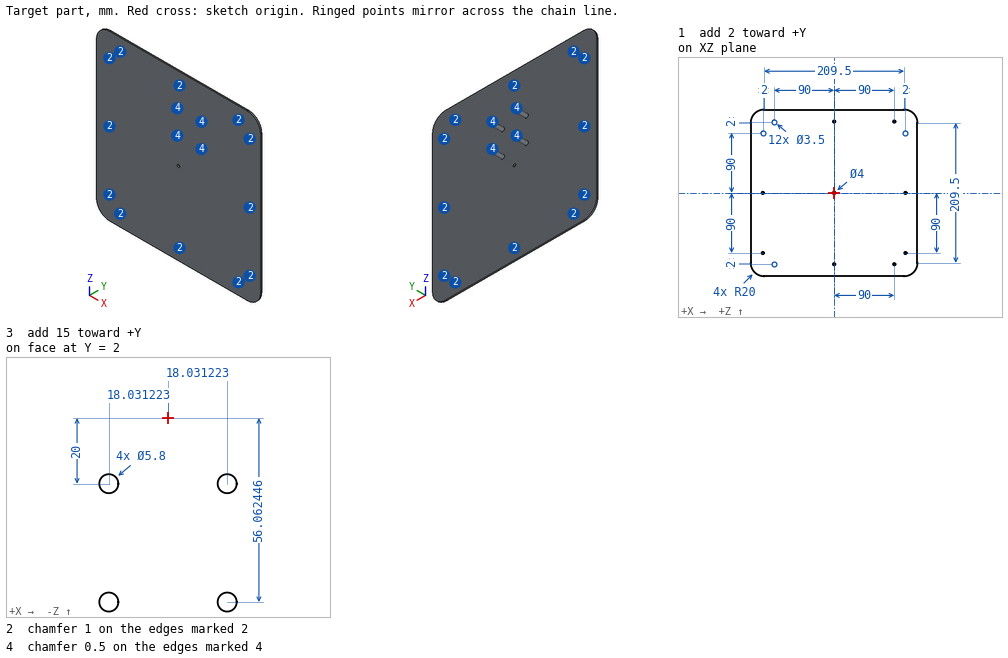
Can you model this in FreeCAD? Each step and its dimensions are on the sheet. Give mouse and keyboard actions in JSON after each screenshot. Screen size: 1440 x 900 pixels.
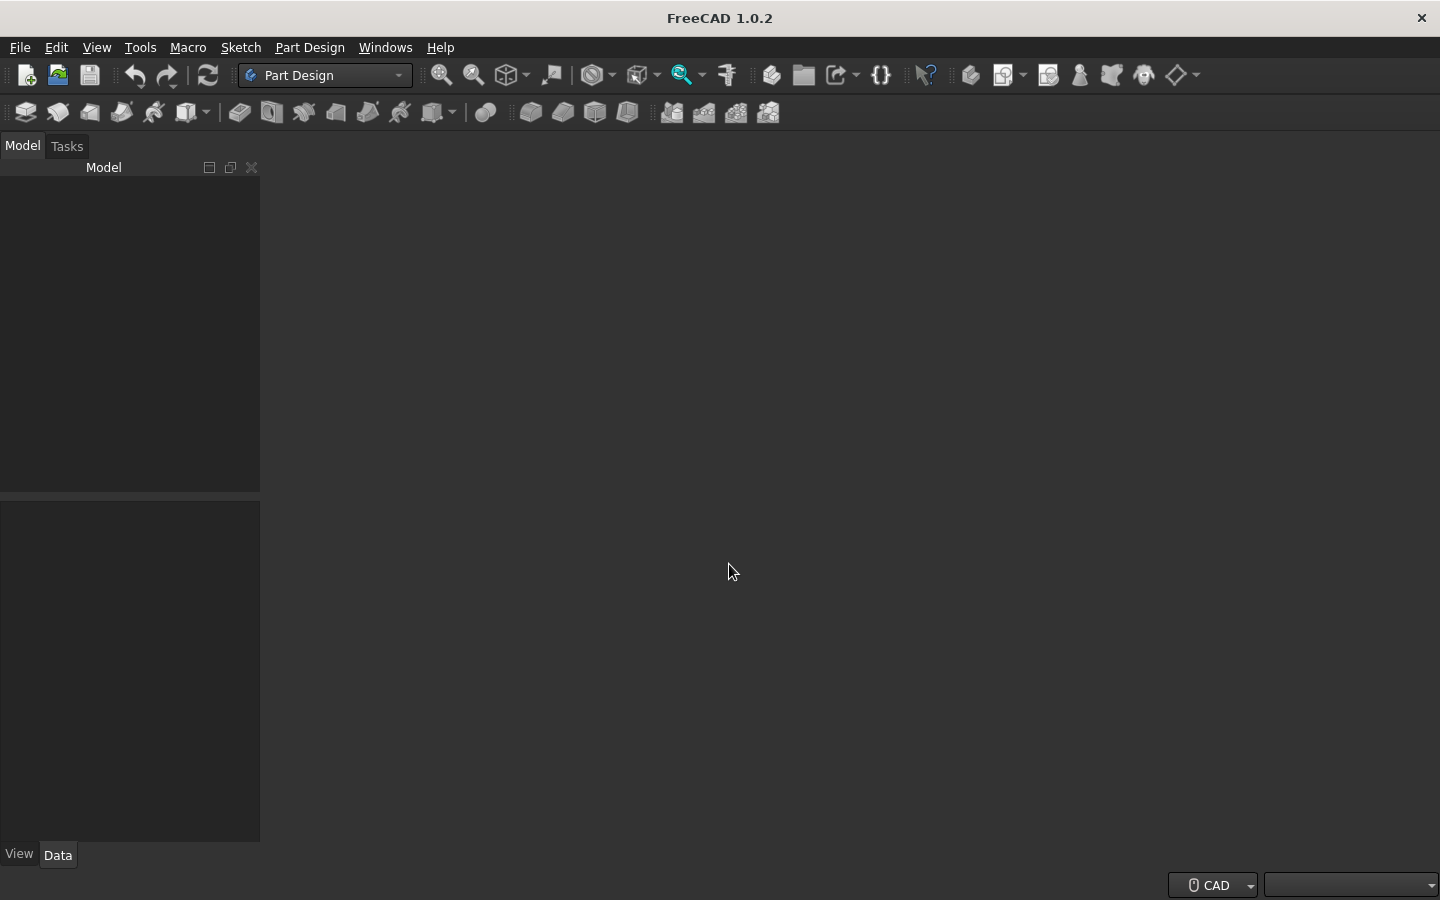
{"action": "left_click", "coordinate": [26, 76]}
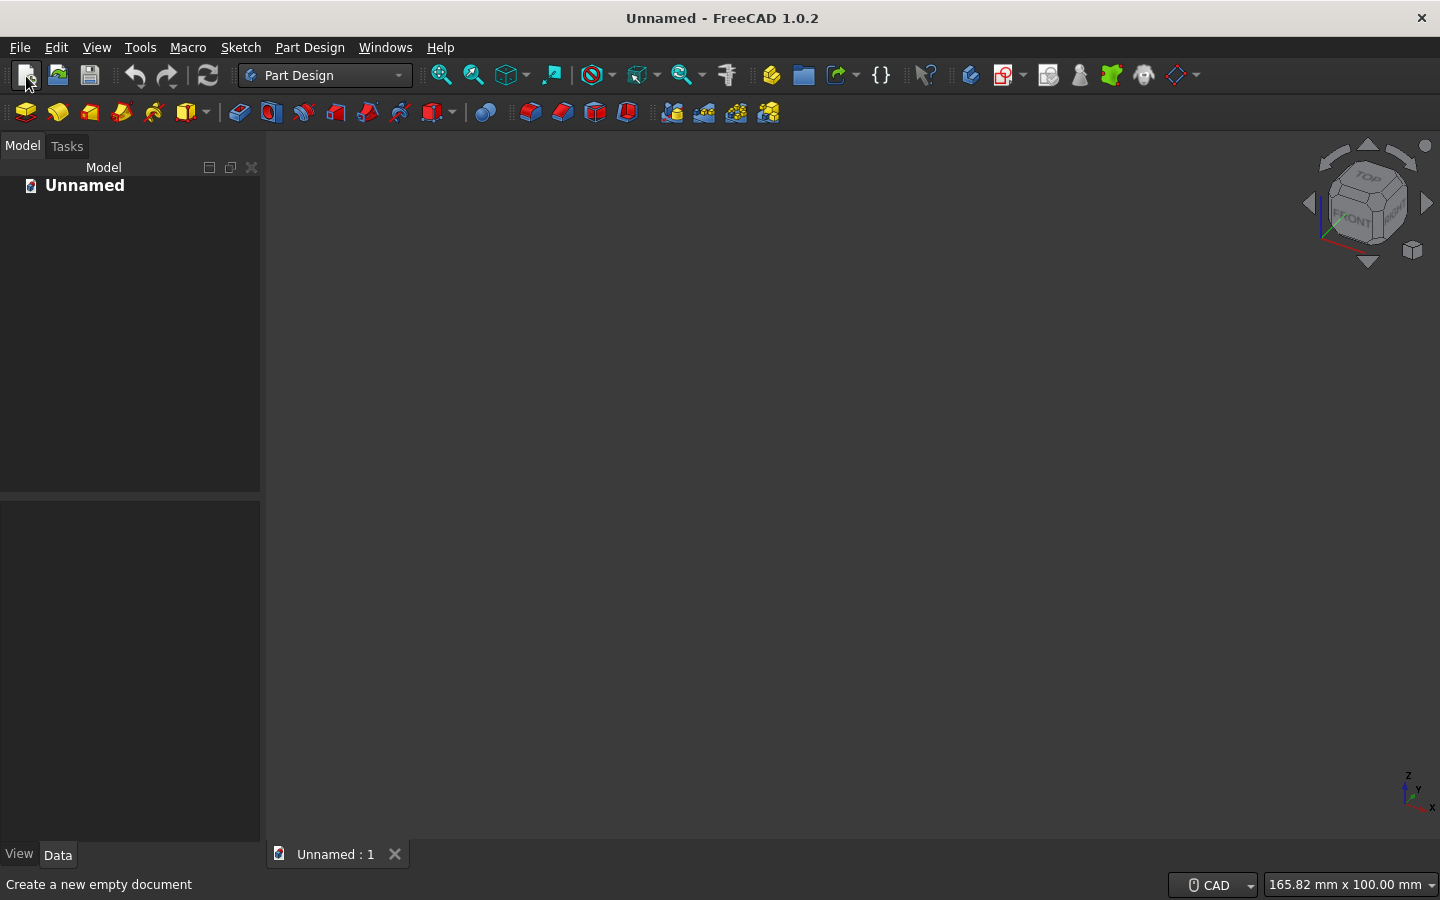
{"action": "left_click", "coordinate": [1004, 76]}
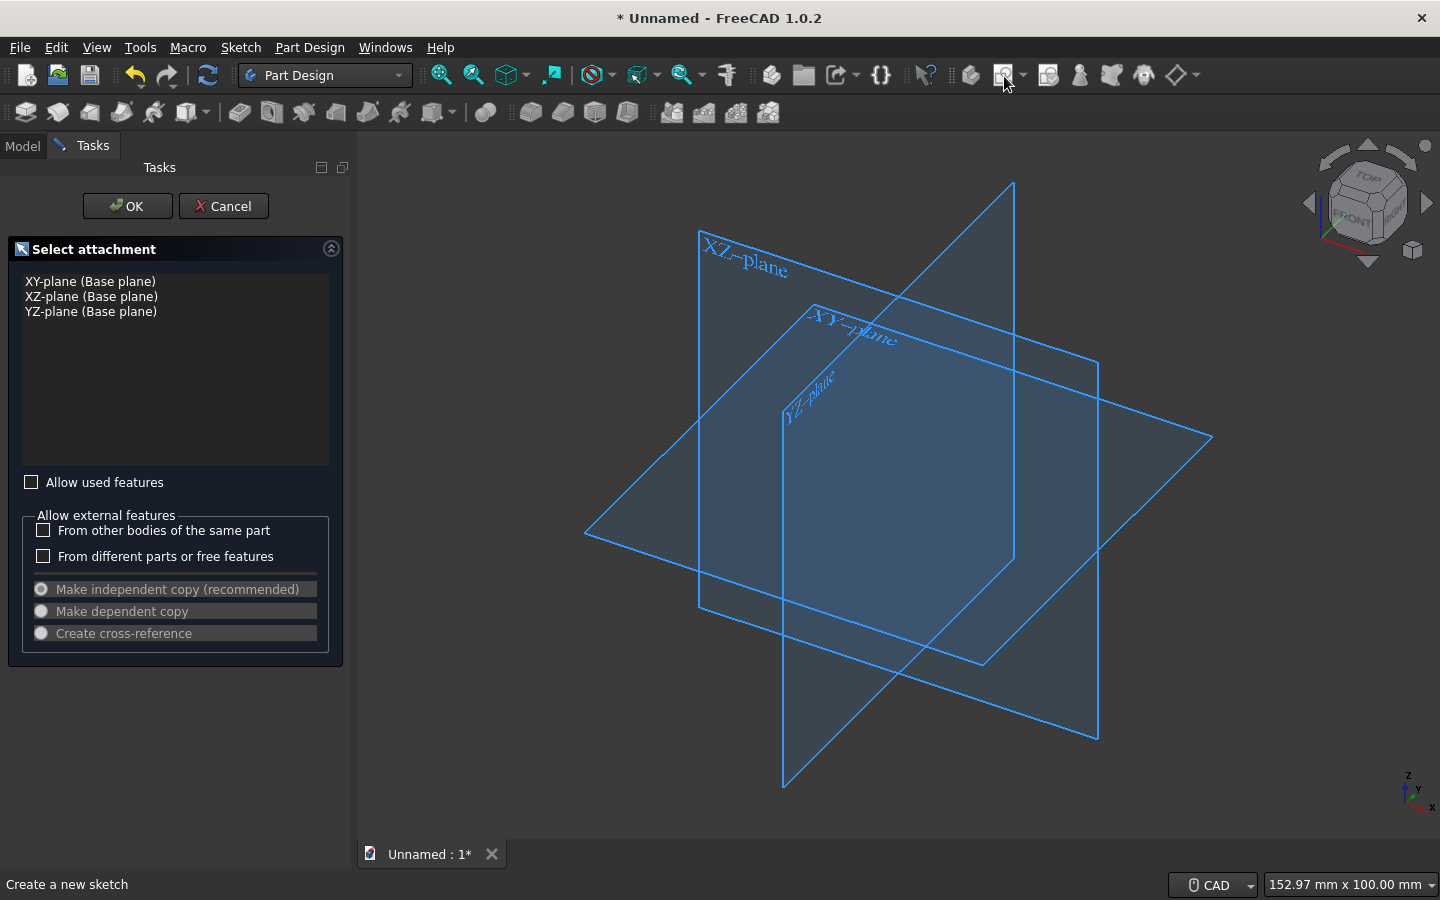
{"action": "left_click", "coordinate": [82, 296]}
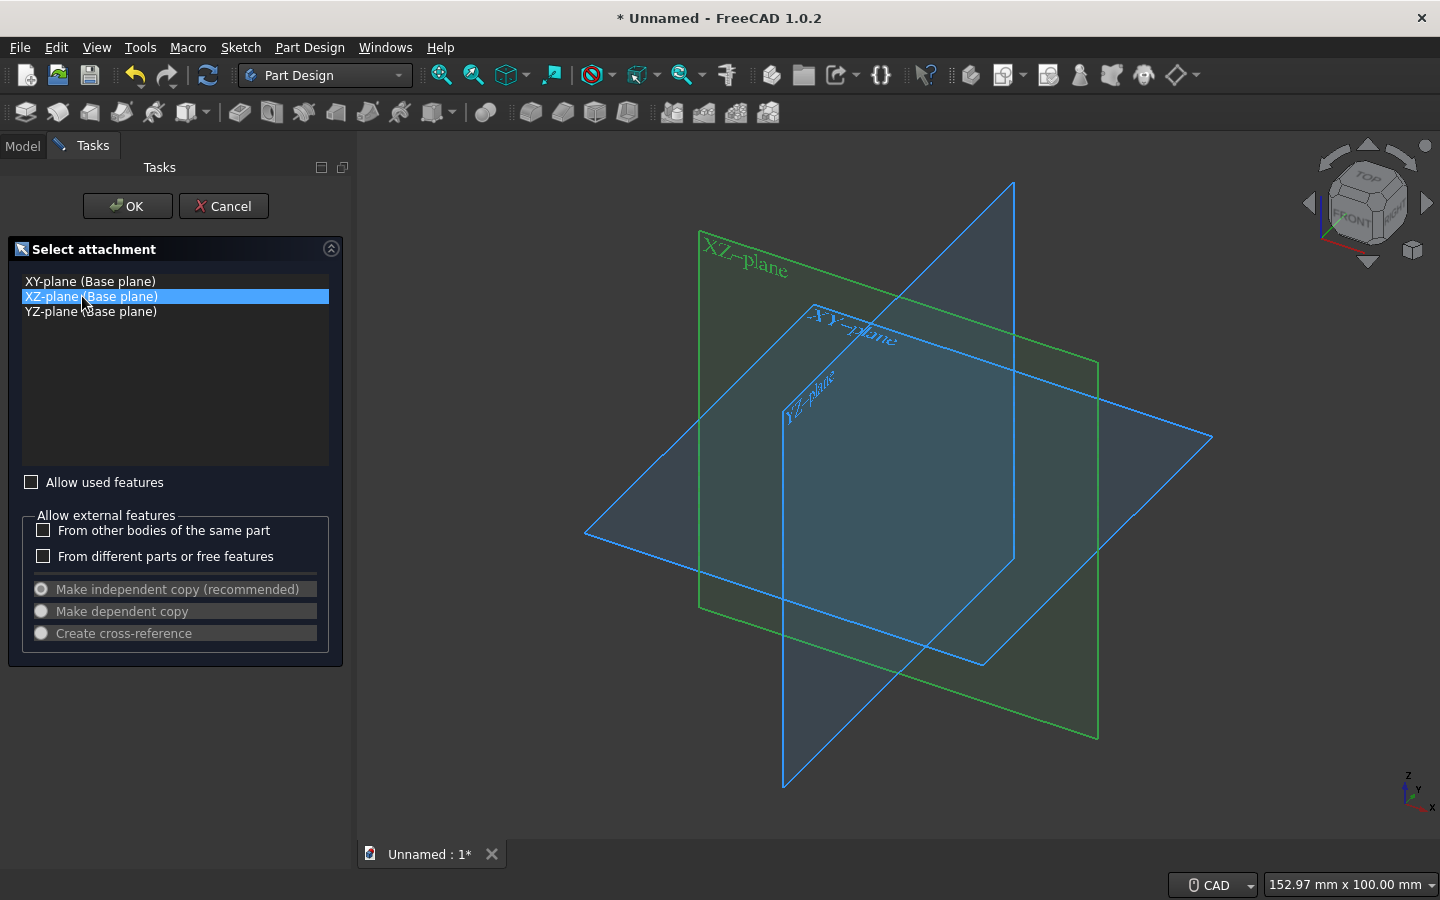
{"action": "left_click", "coordinate": [128, 206]}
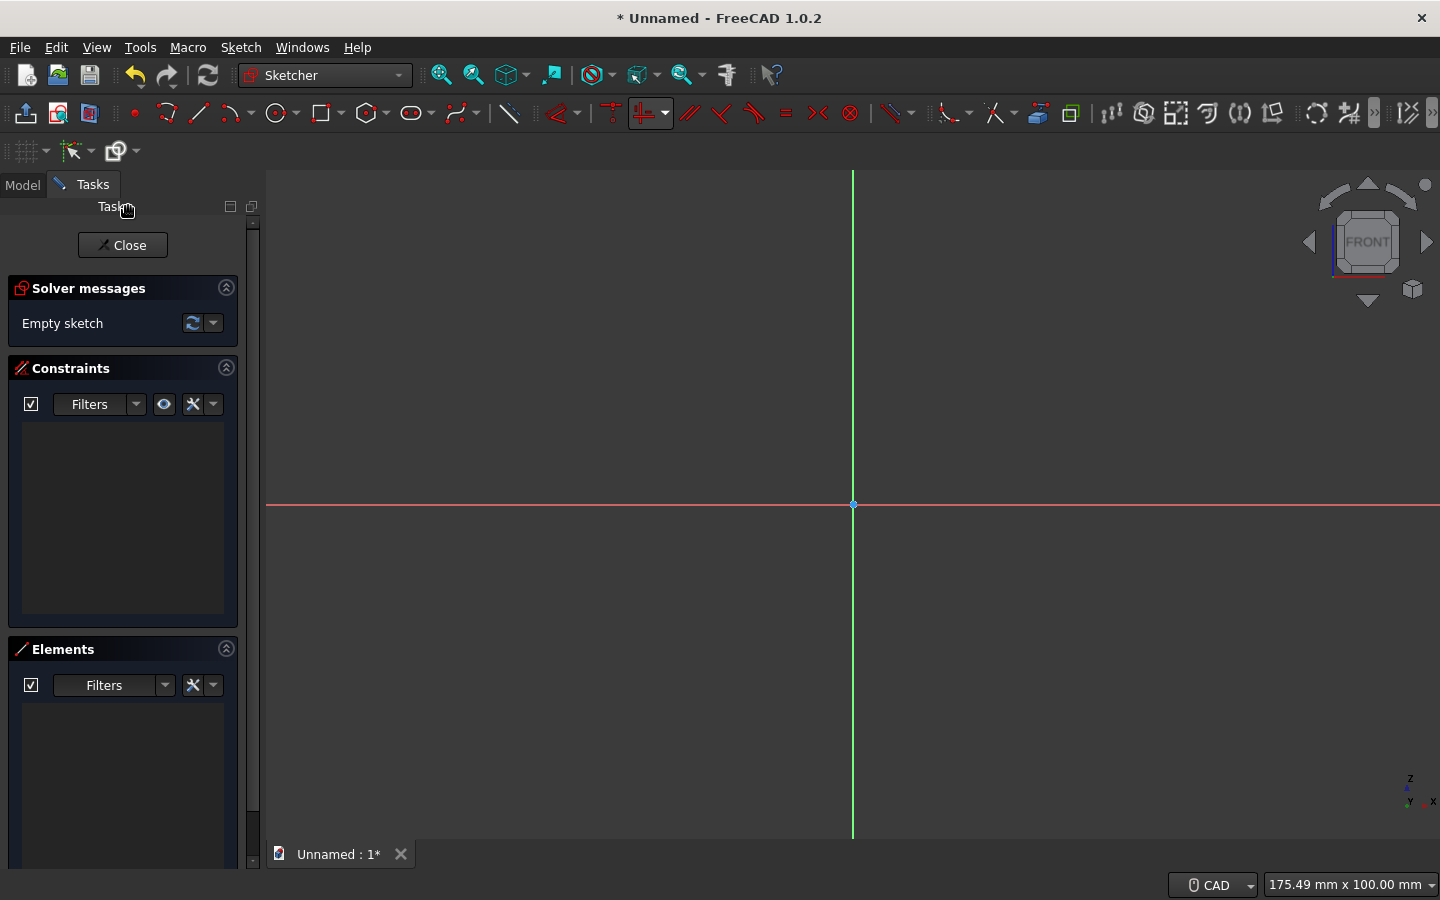
{"action": "scroll", "coordinate": [762, 504], "scroll_direction": "down", "scroll_amount": 7}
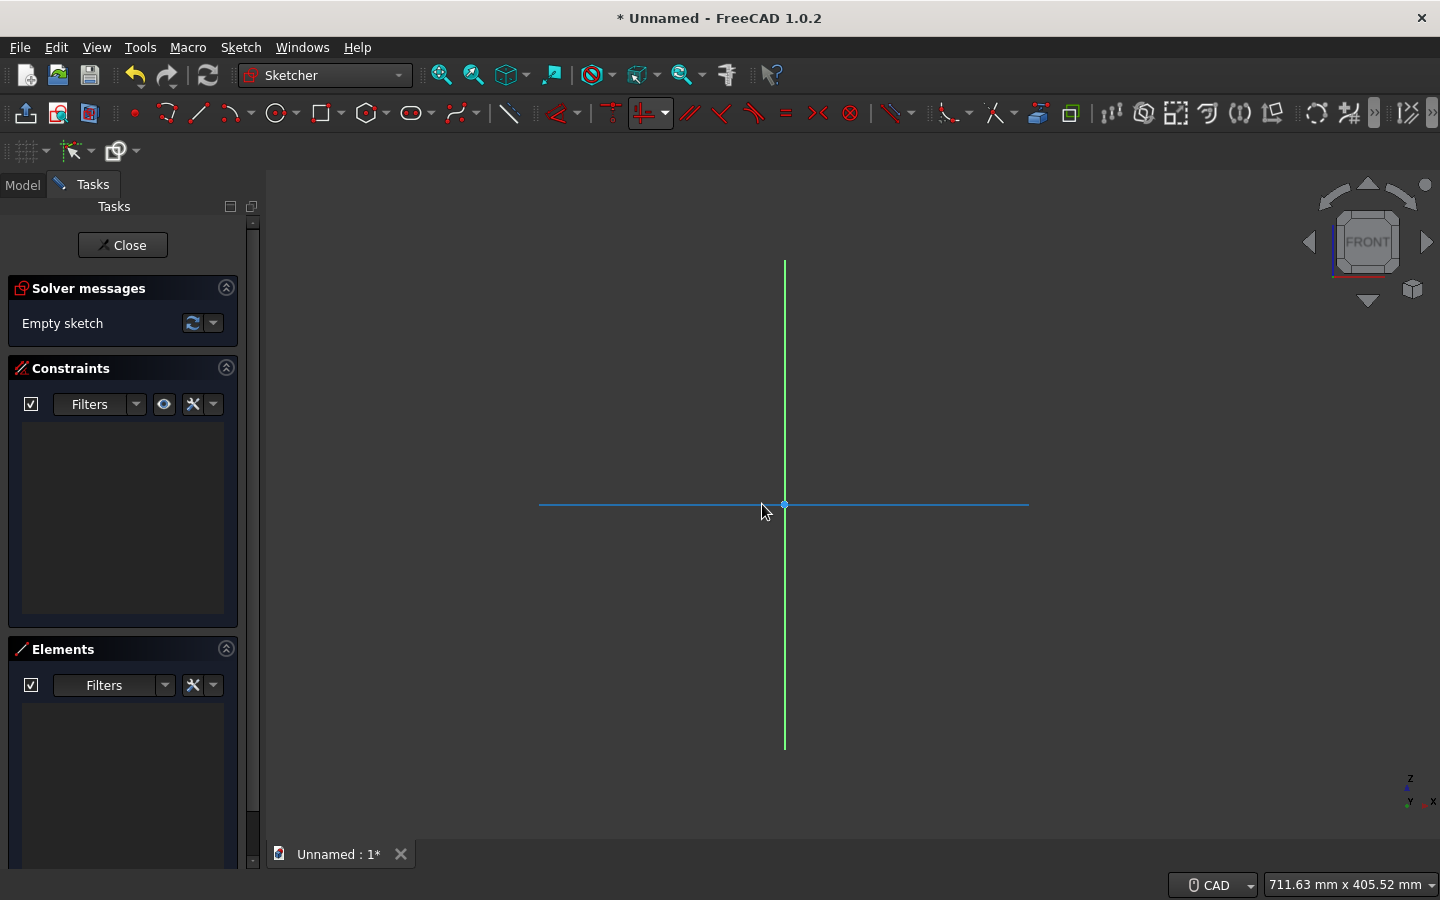
{"action": "key", "text": "g l"}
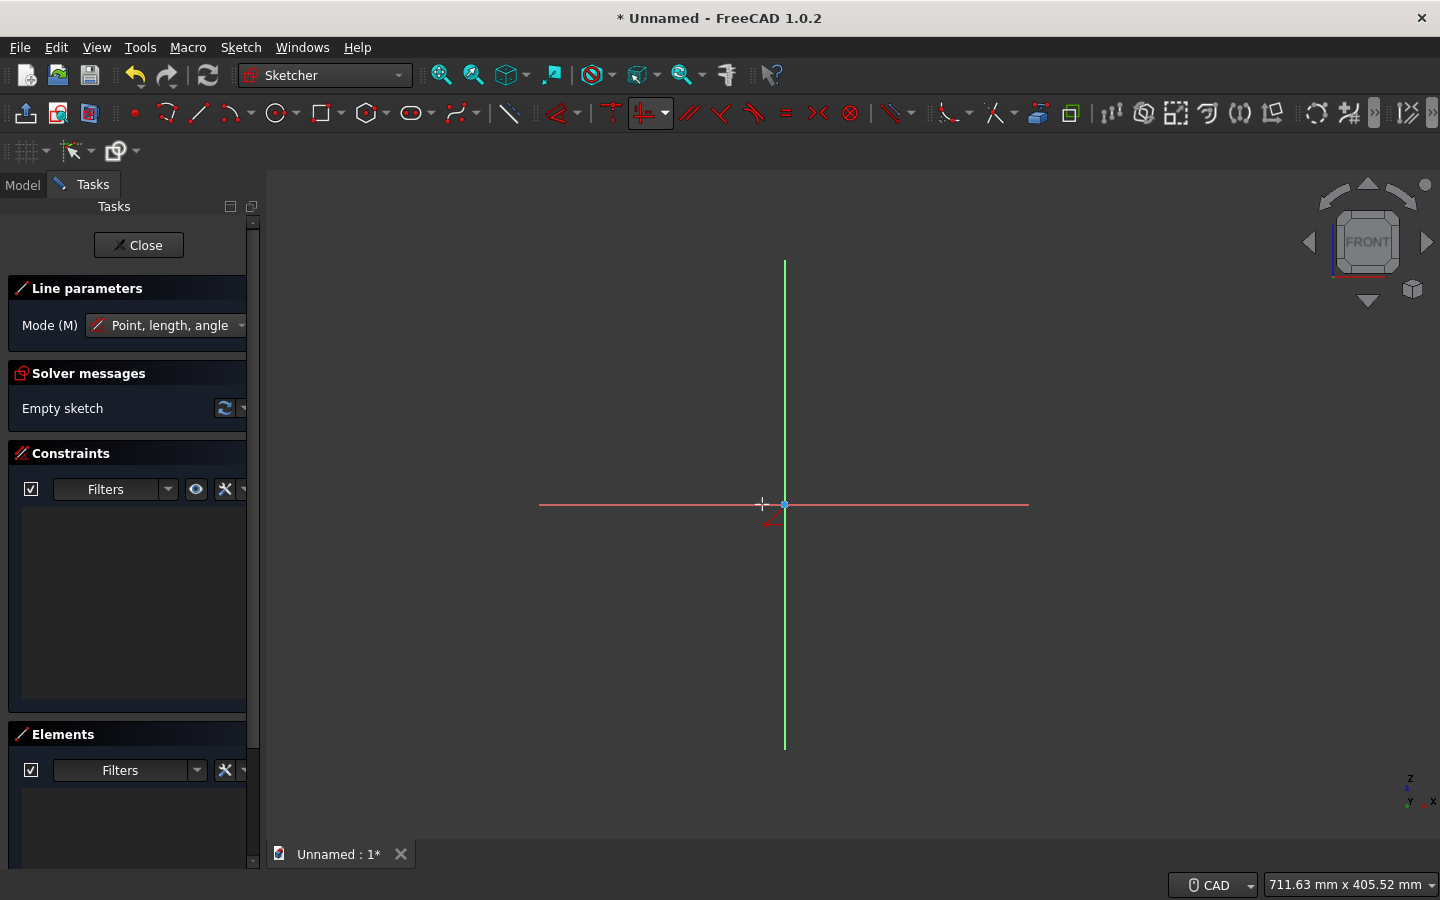
{"action": "left_click", "coordinate": [612, 299]}
{"action": "left_click", "coordinate": [958, 299]}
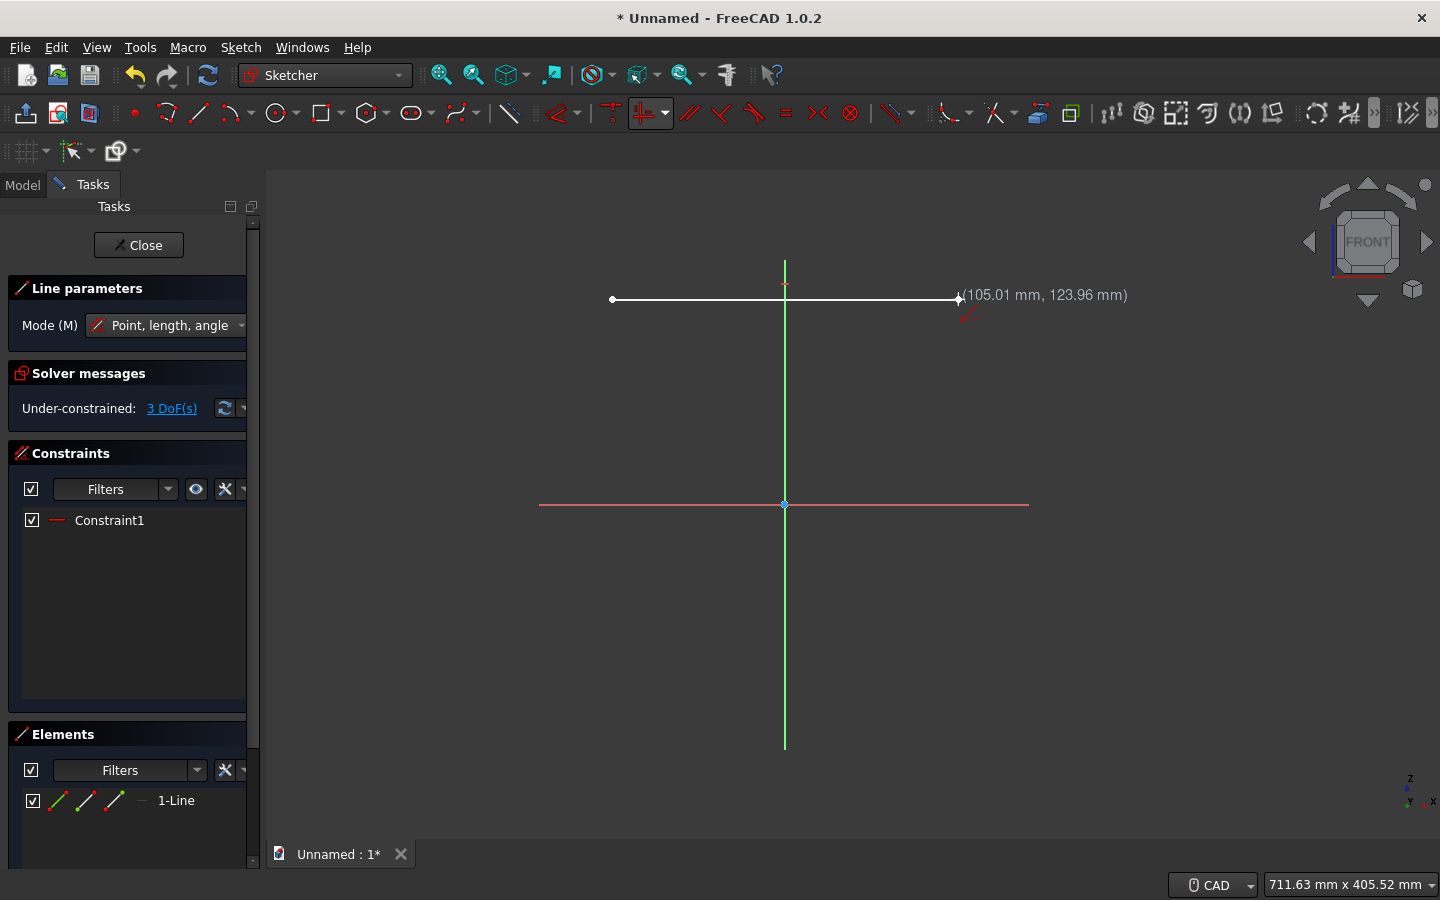
{"action": "left_click", "coordinate": [991, 332]}
{"action": "left_click", "coordinate": [991, 677]}